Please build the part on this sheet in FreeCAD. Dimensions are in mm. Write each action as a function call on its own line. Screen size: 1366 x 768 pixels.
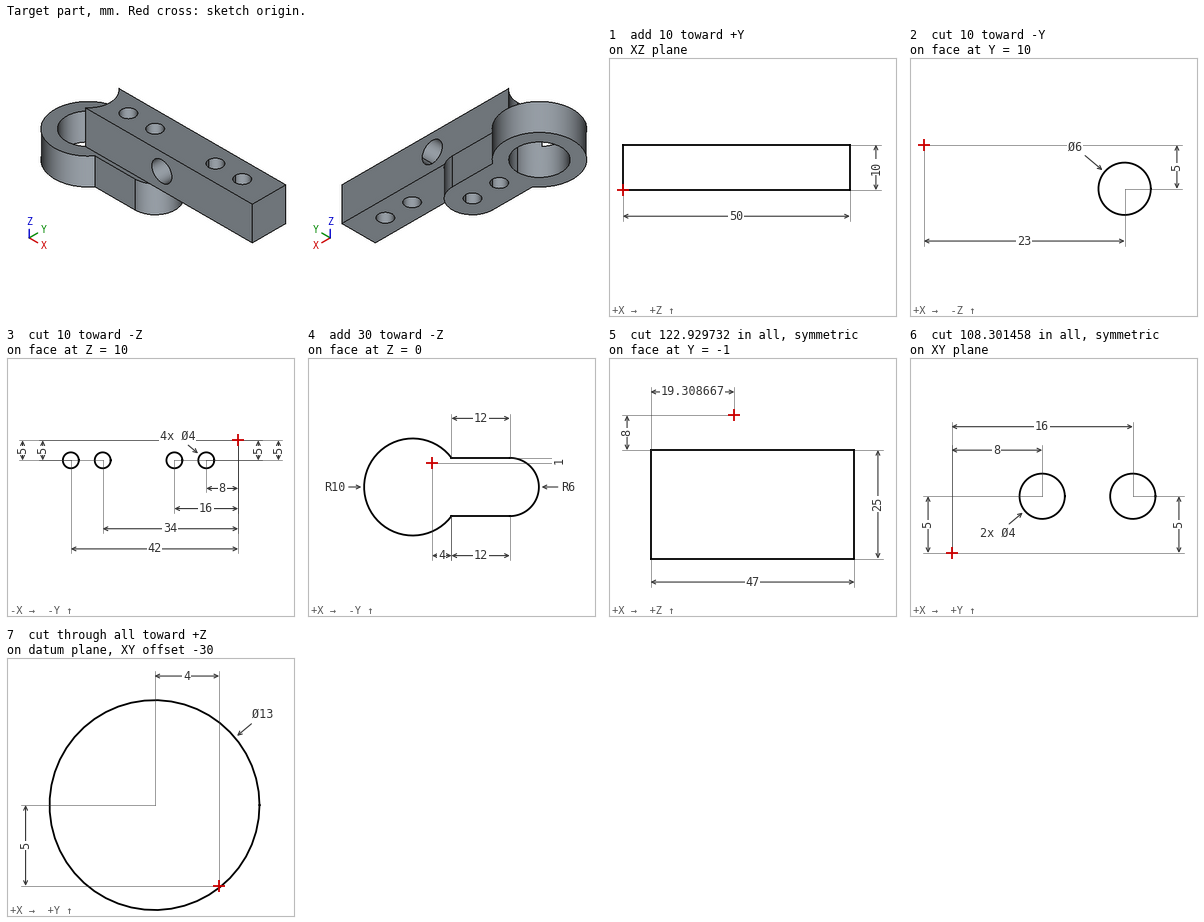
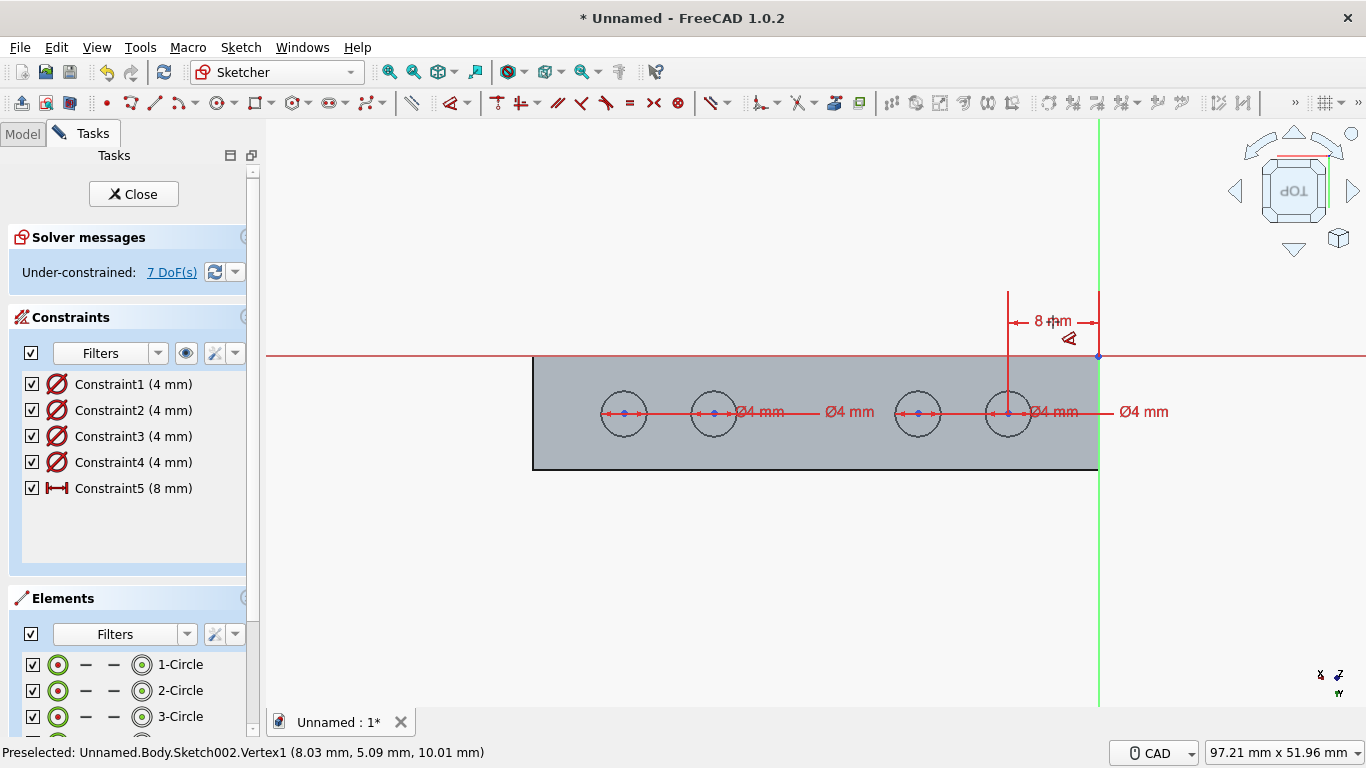
click(1008, 414)
click(1133, 385)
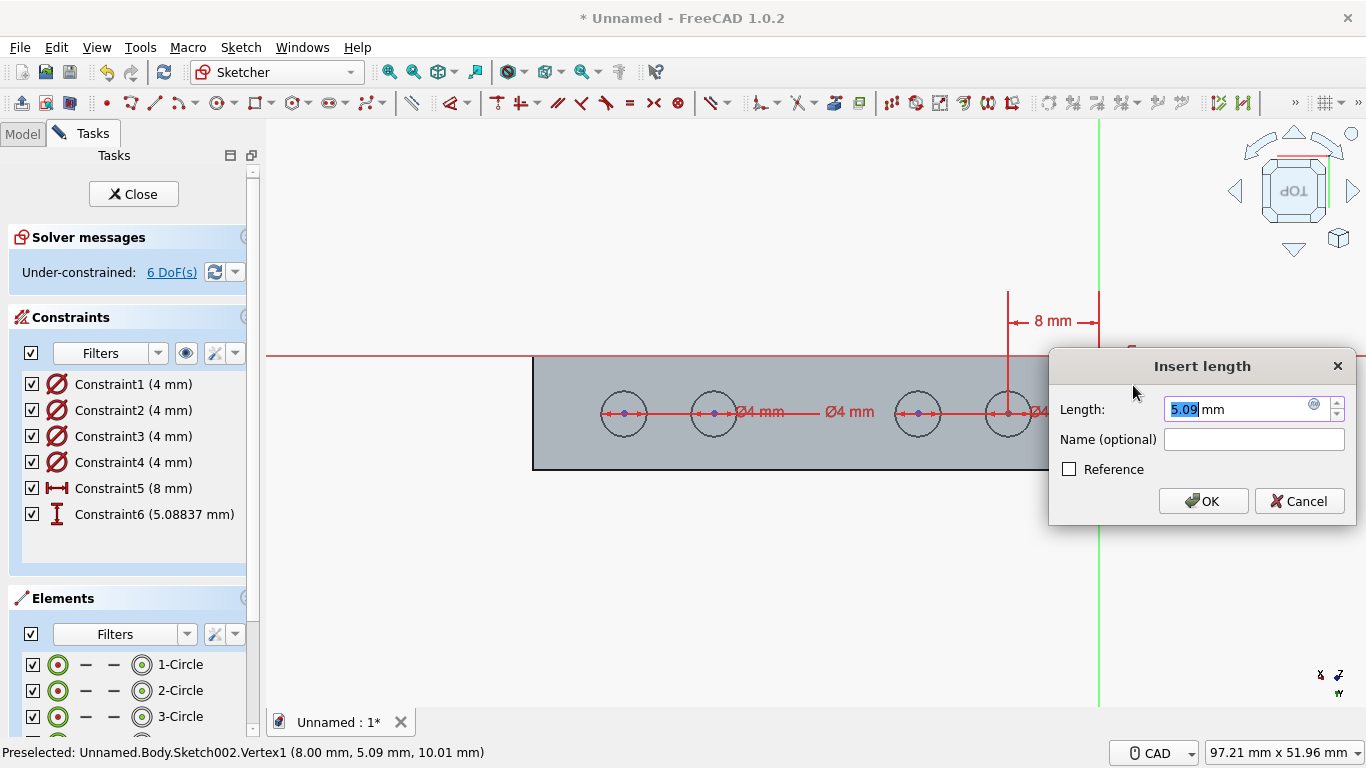
text(5)
key(Return)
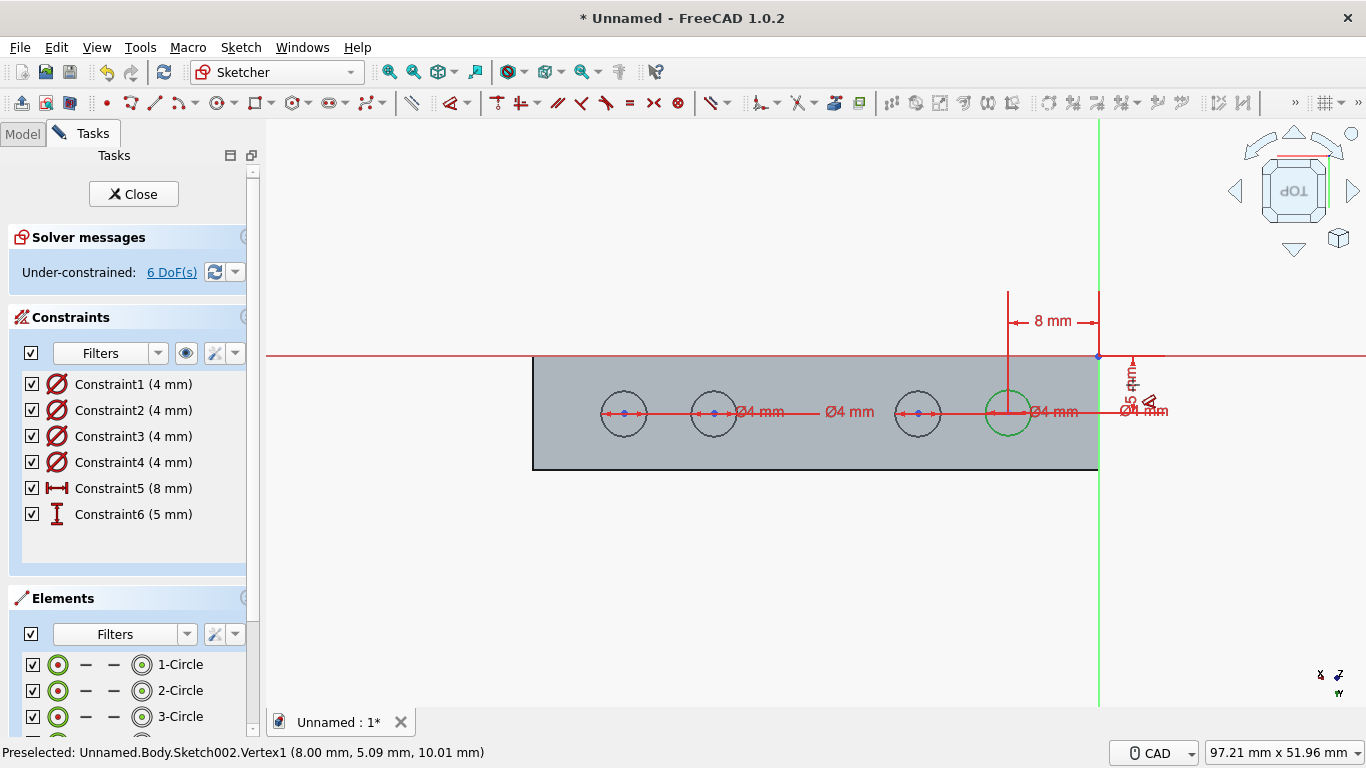
click(918, 414)
click(1133, 405)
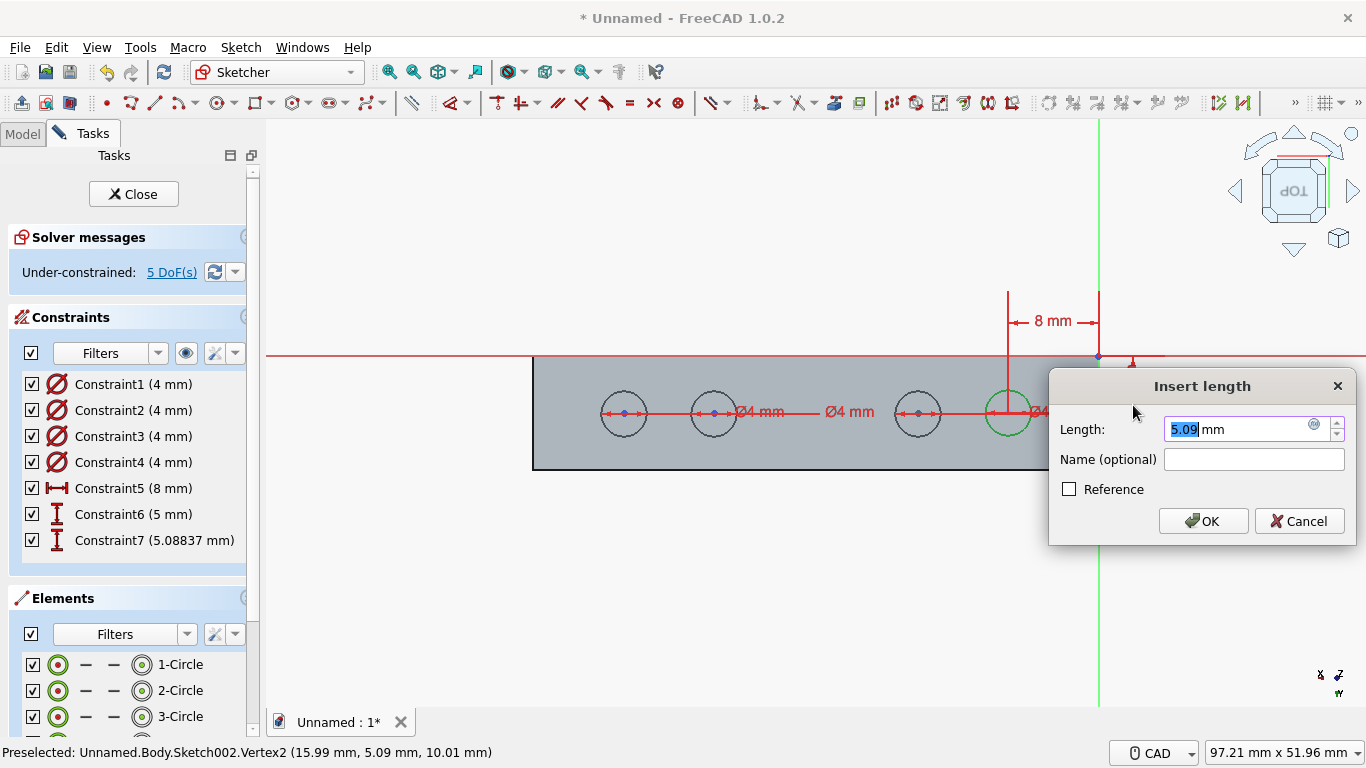
text(5)
key(Return)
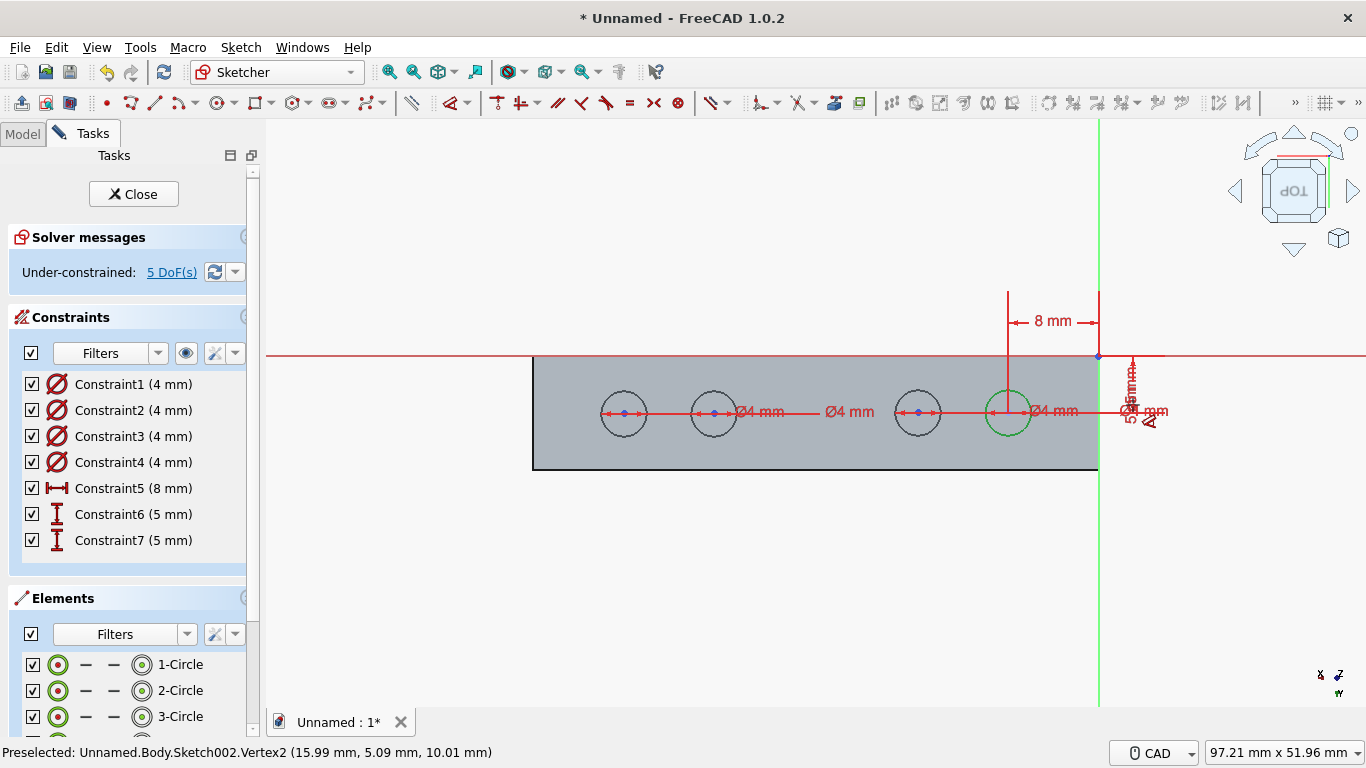
click(624, 414)
click(590, 385)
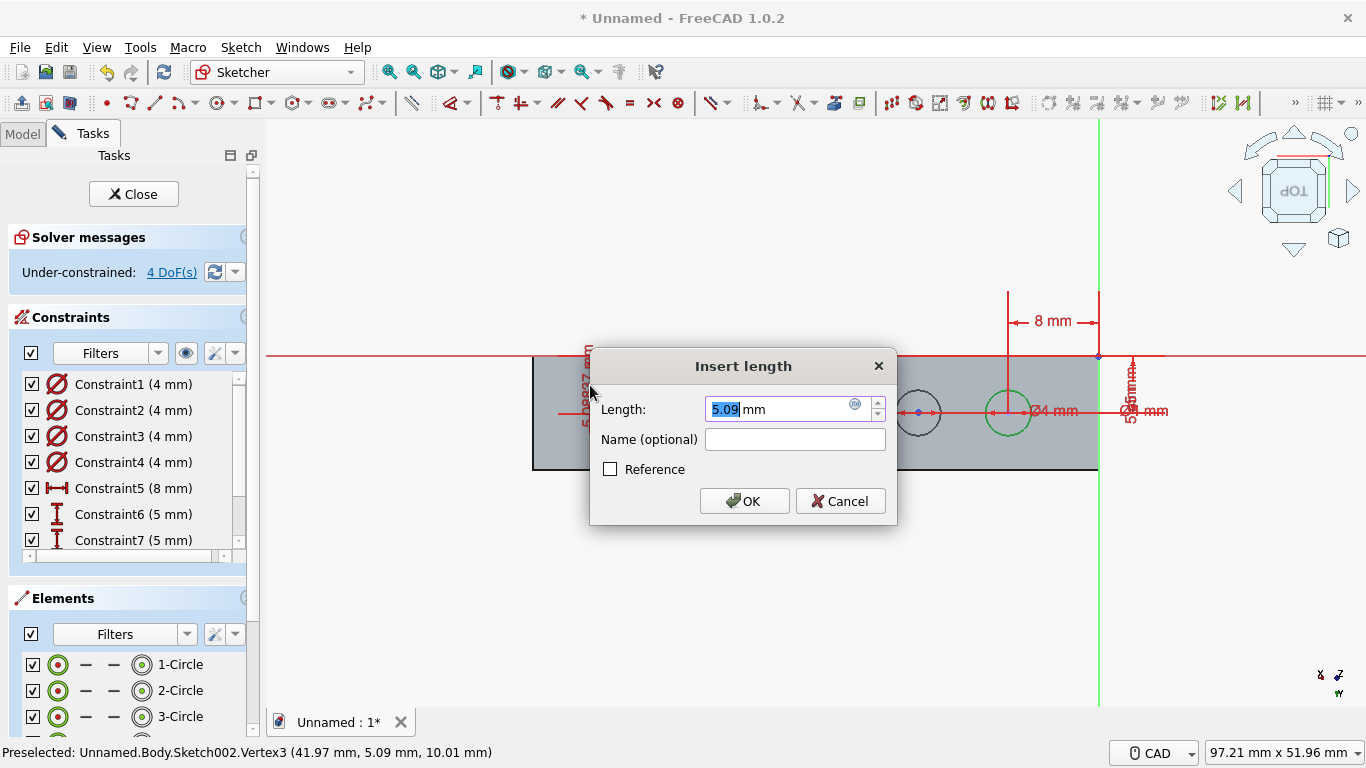
text(5)
key(Return)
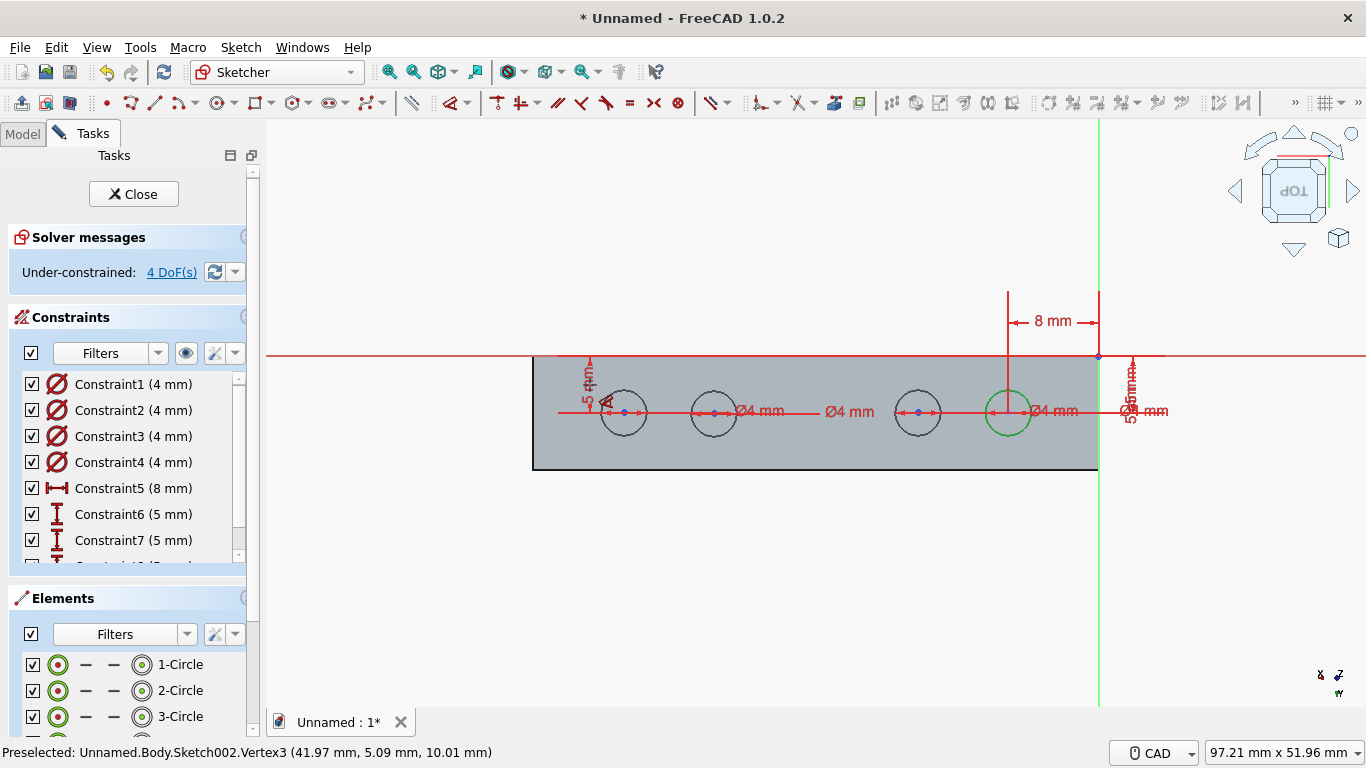
click(714, 414)
click(680, 385)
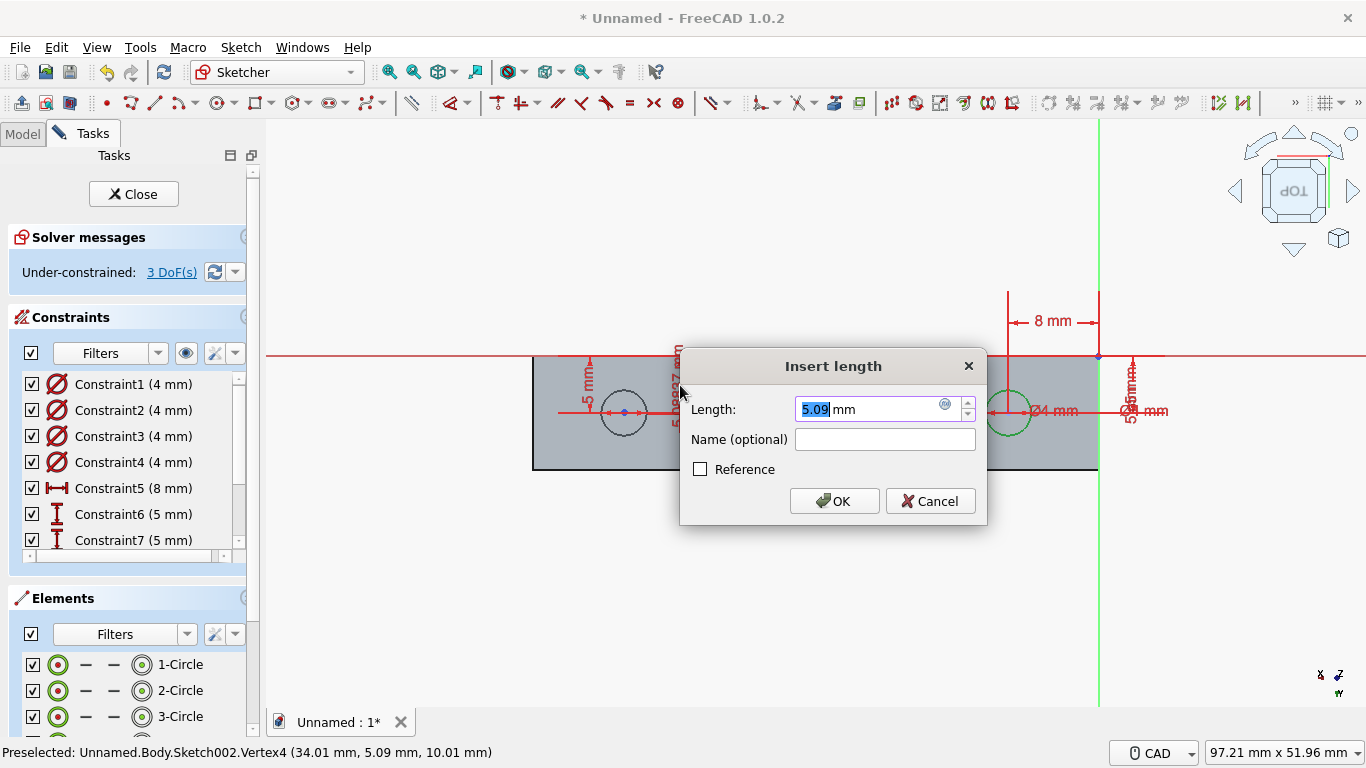
text(5)
key(Return)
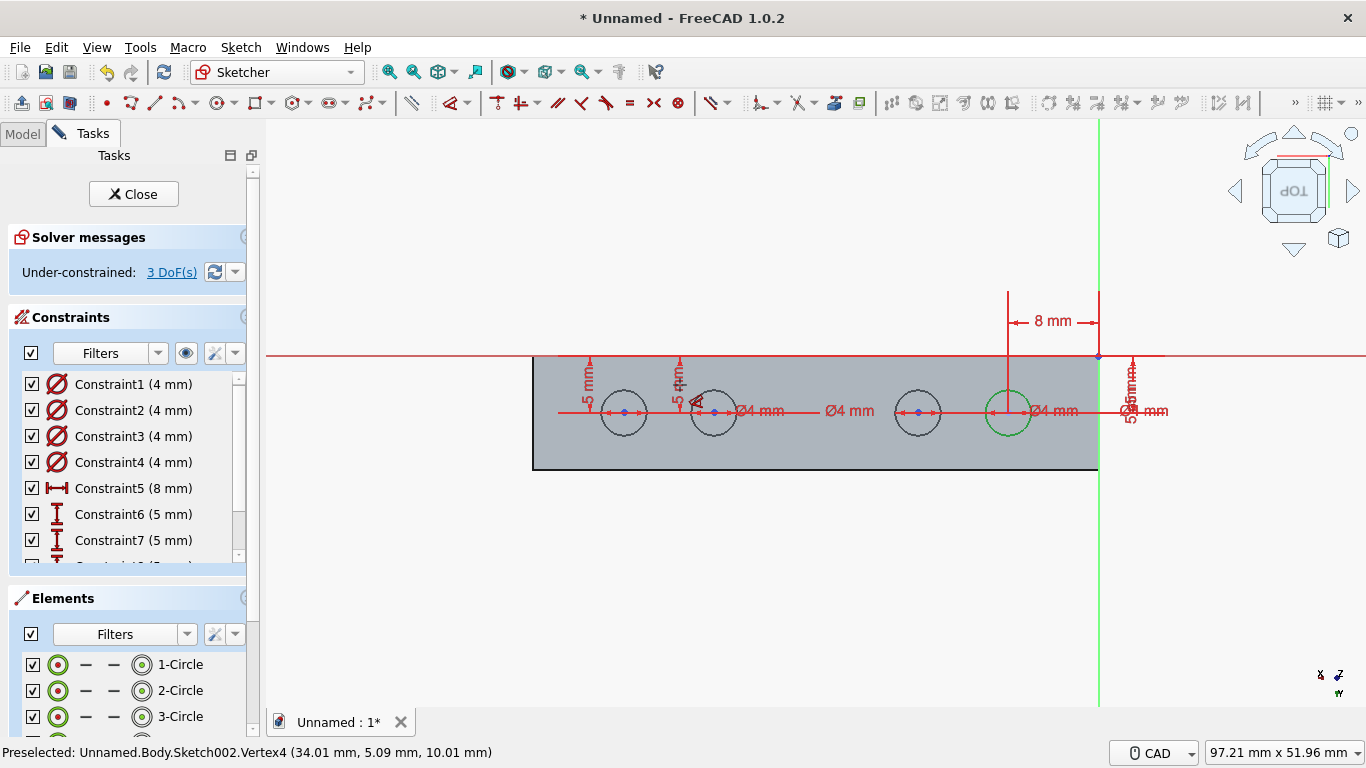
click(918, 413)
click(967, 322)